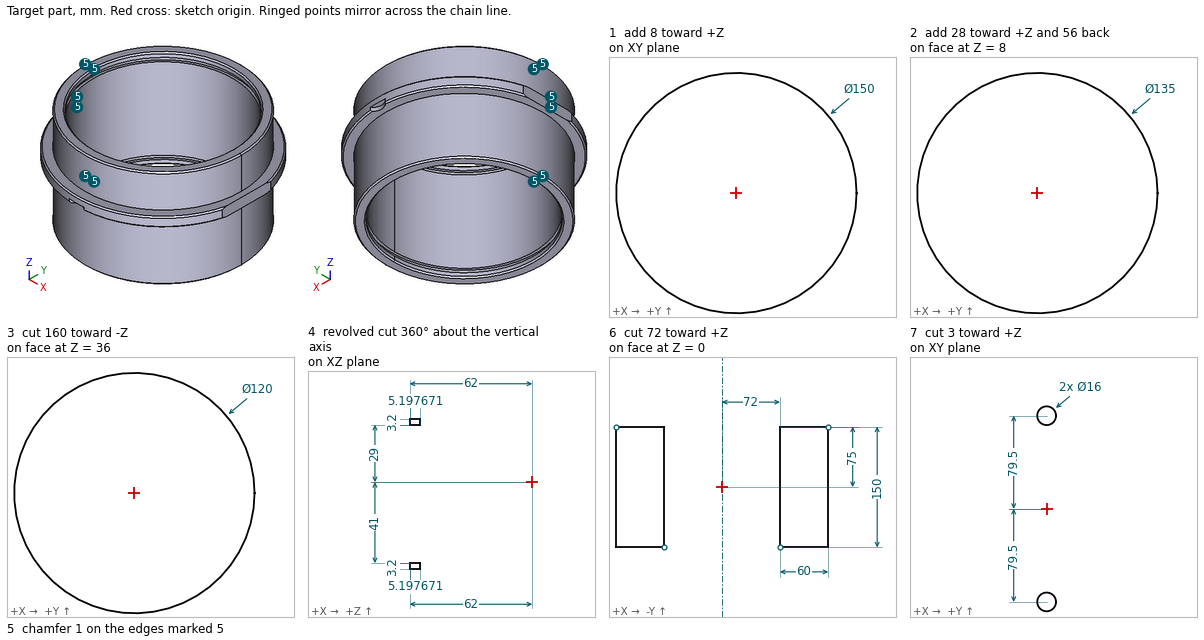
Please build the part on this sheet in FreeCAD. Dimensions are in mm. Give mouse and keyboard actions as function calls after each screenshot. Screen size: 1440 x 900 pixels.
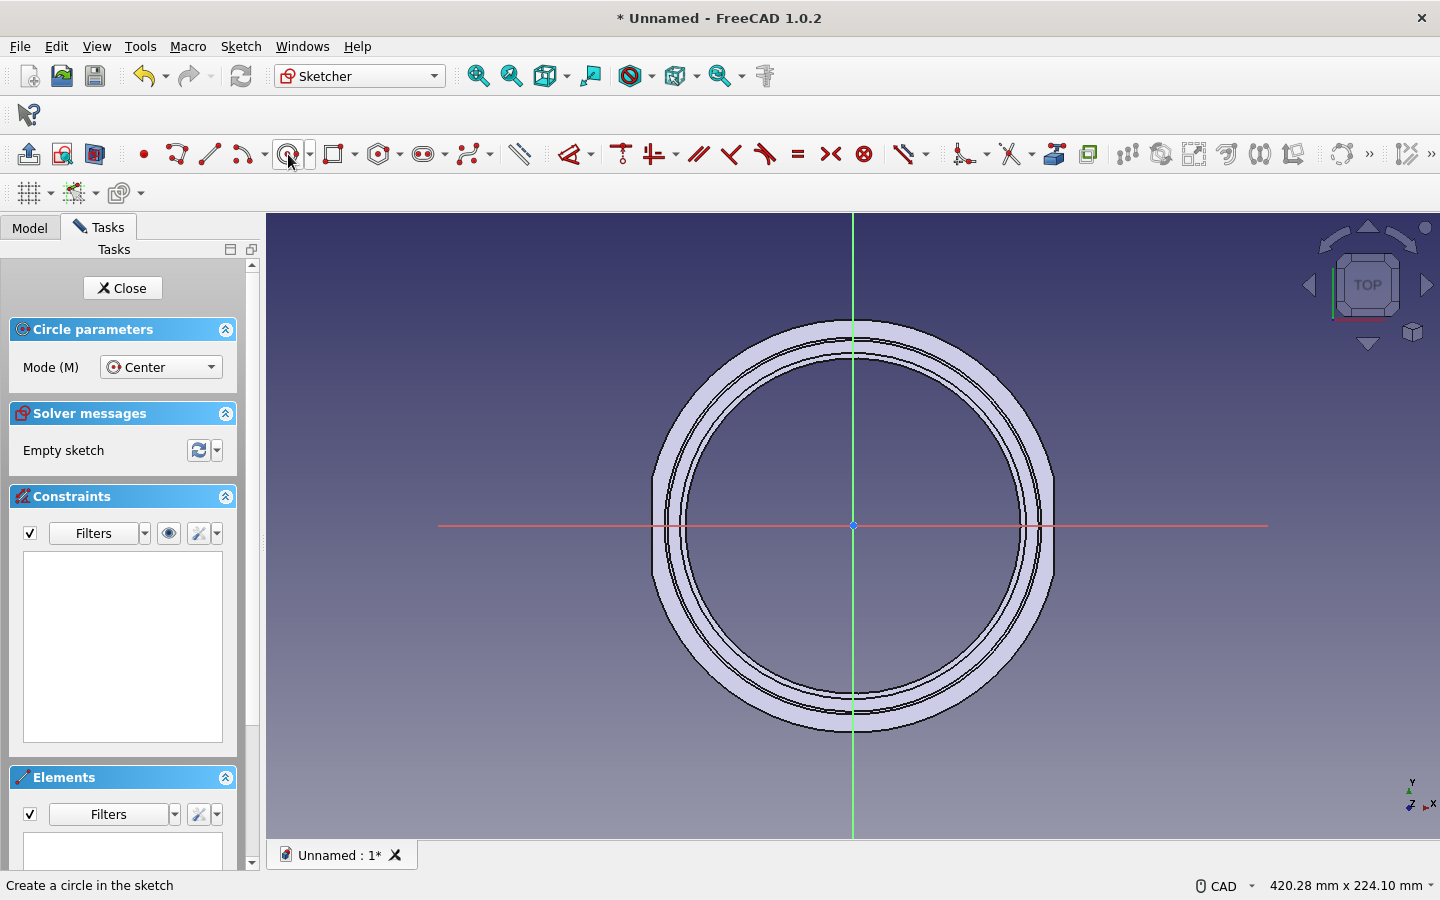
click(853, 304)
click(869, 288)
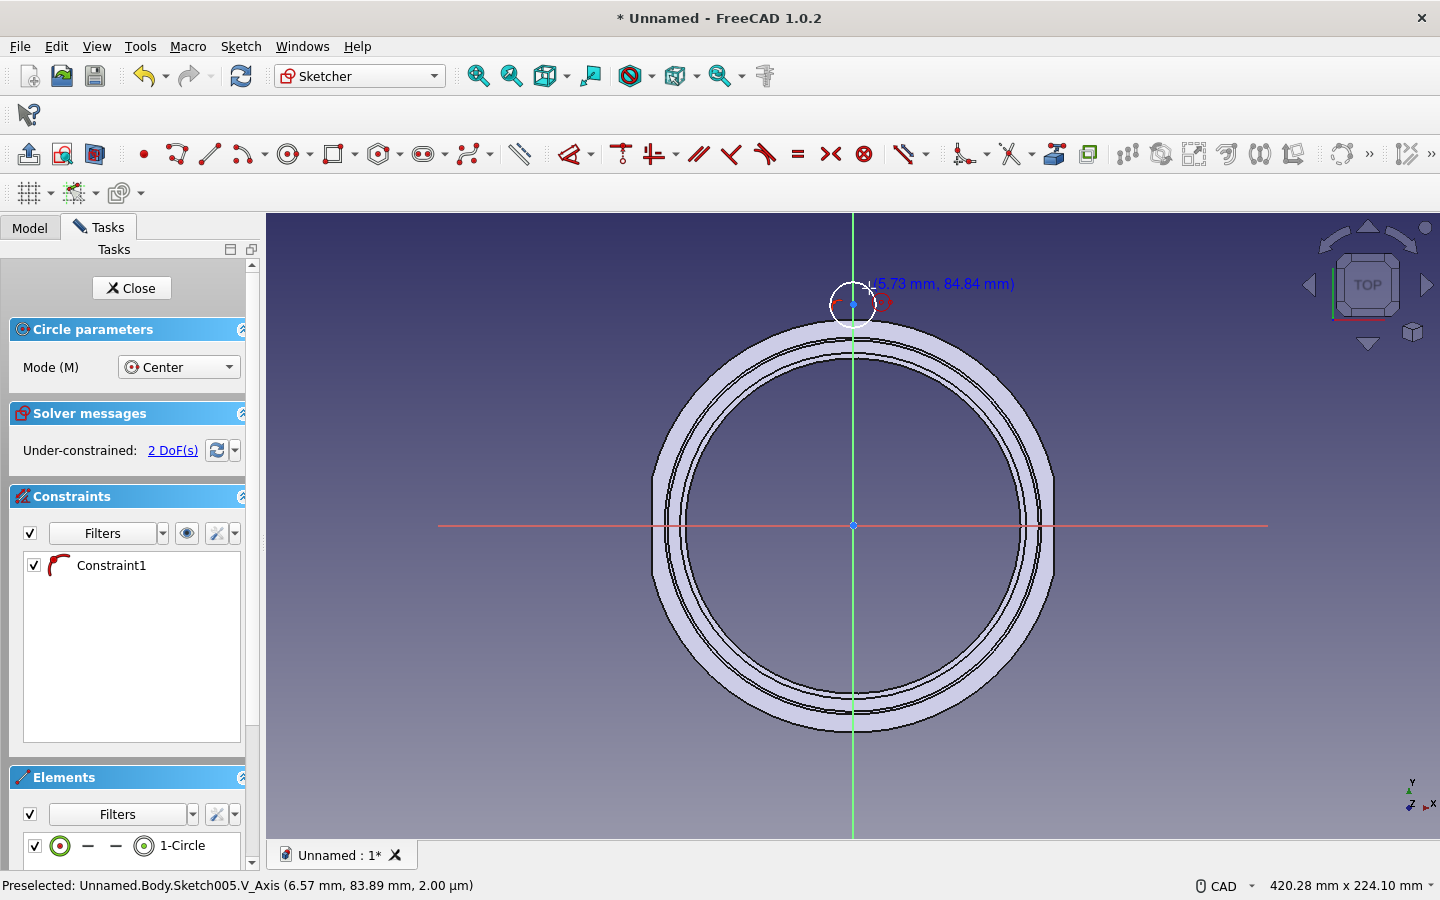
click(853, 748)
click(869, 732)
key(Escape)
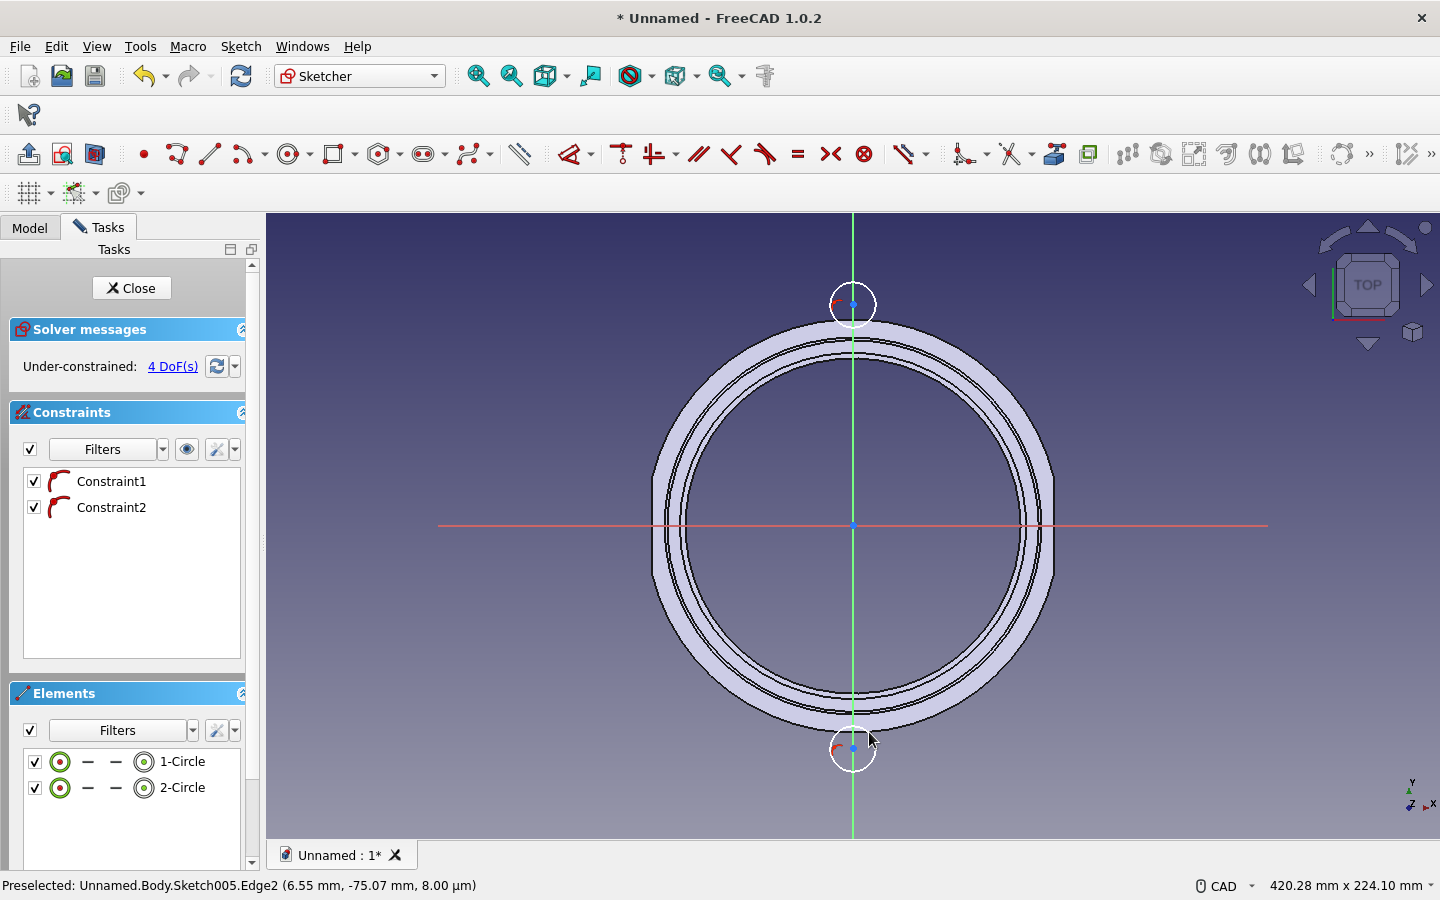
click(869, 289)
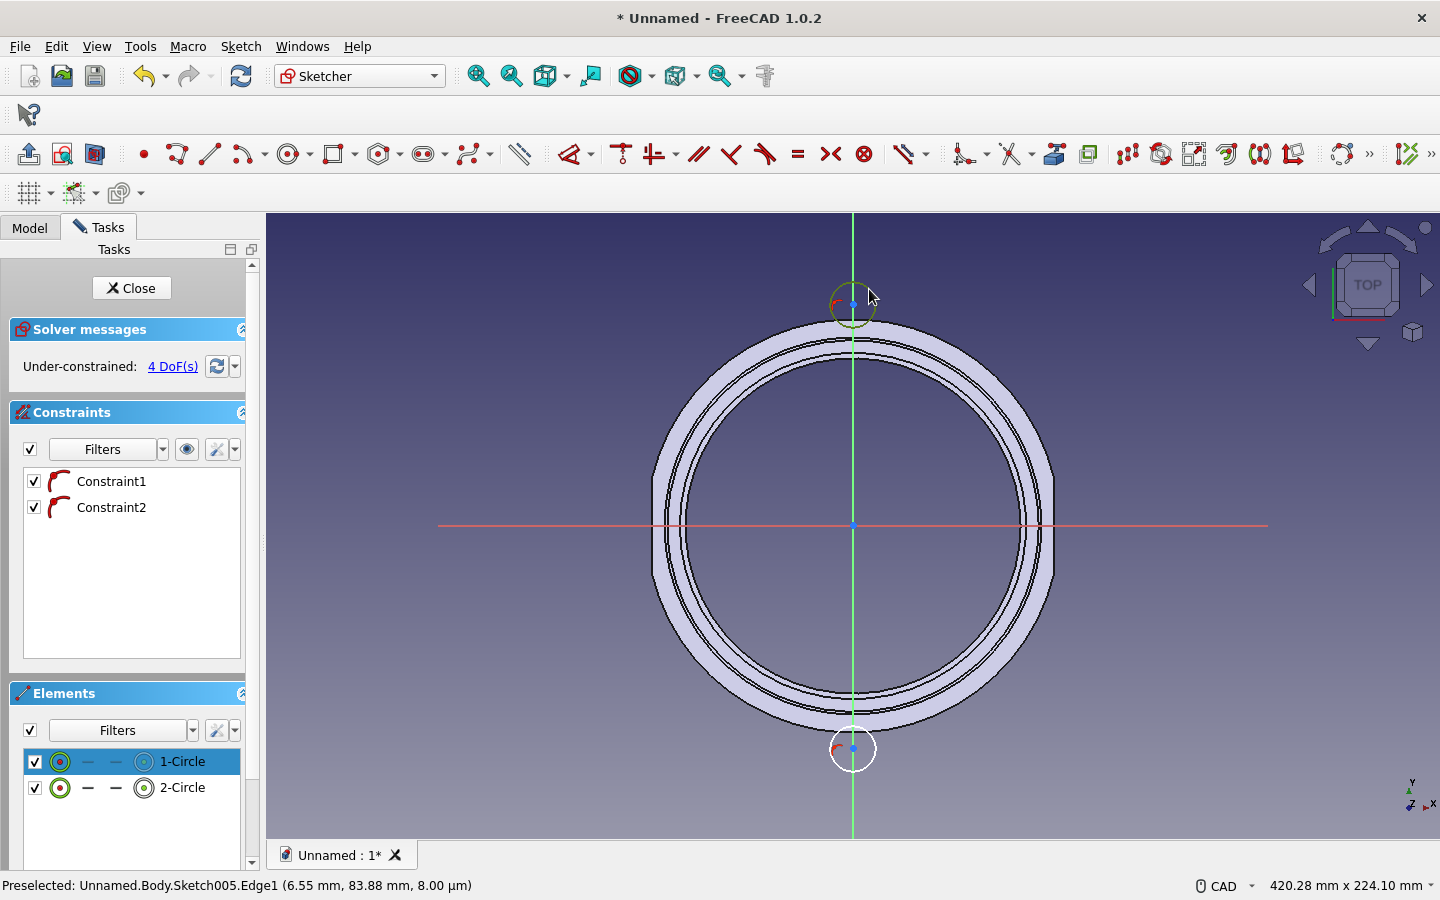
click(869, 733)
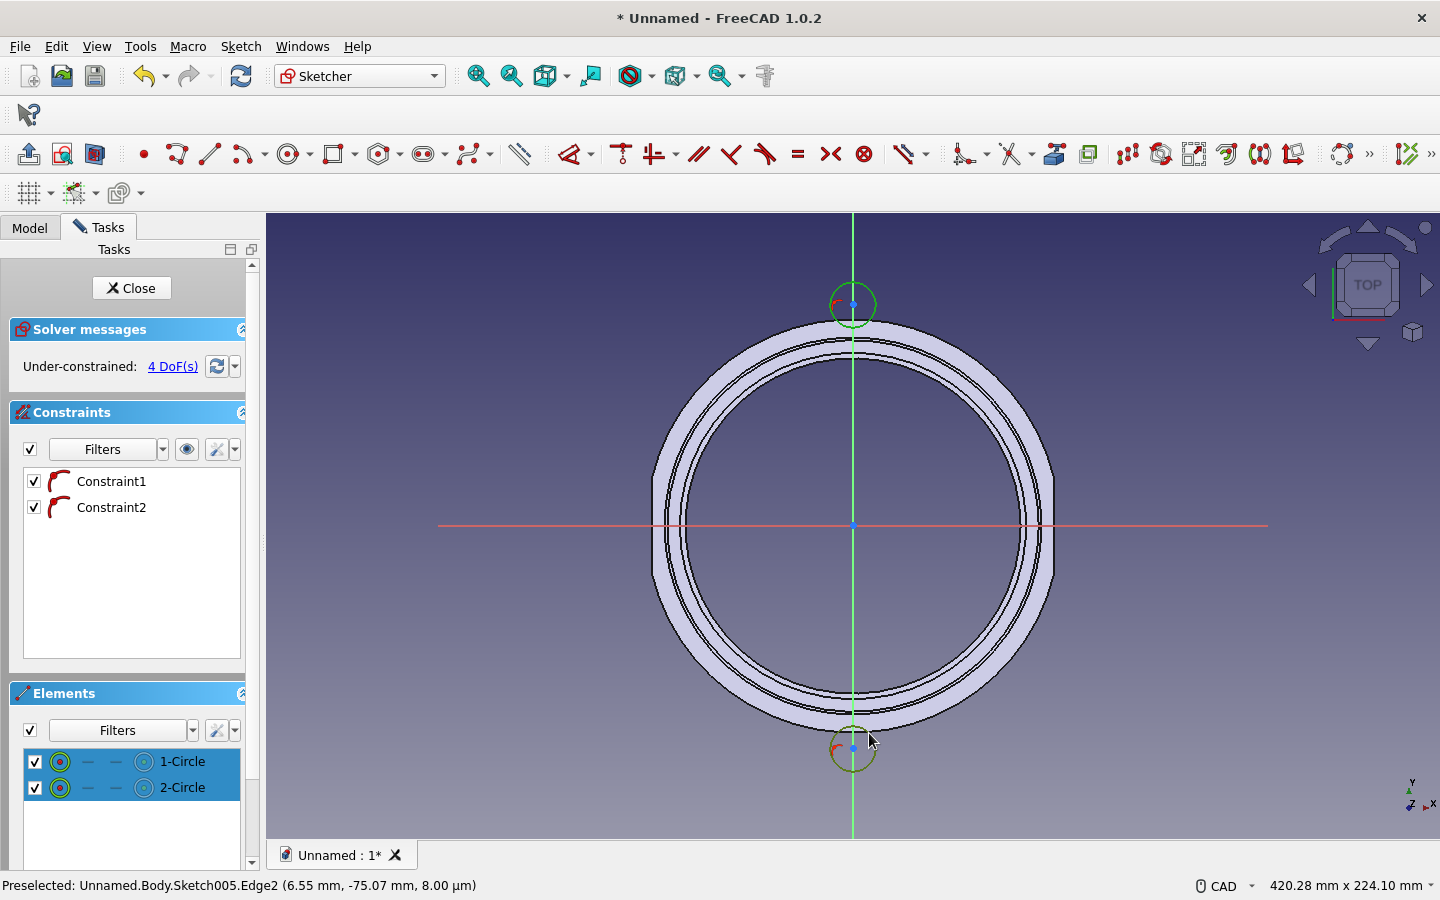
key(e)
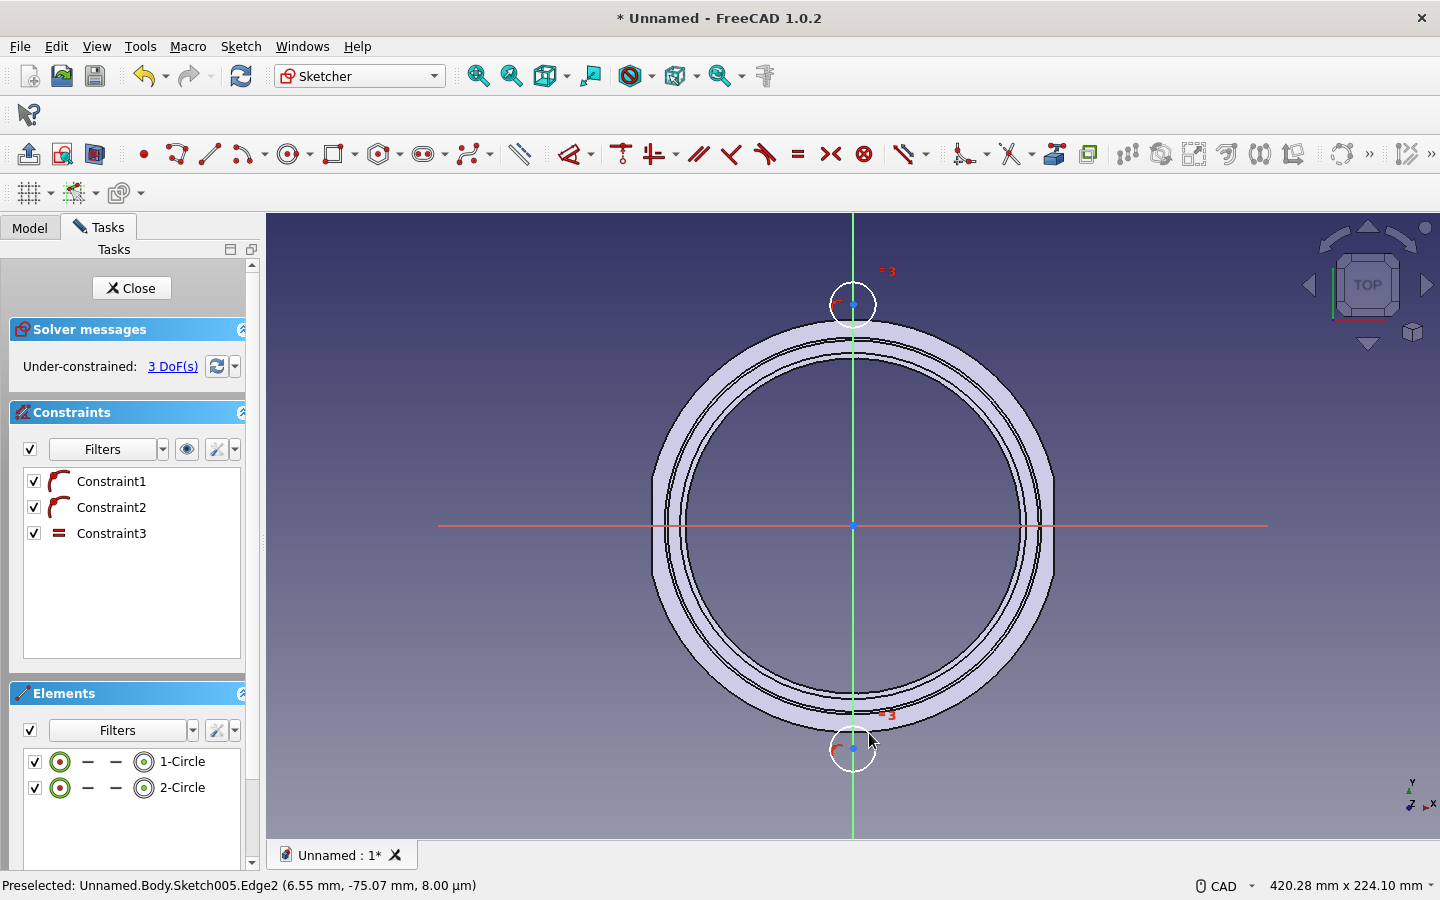
click(568, 154)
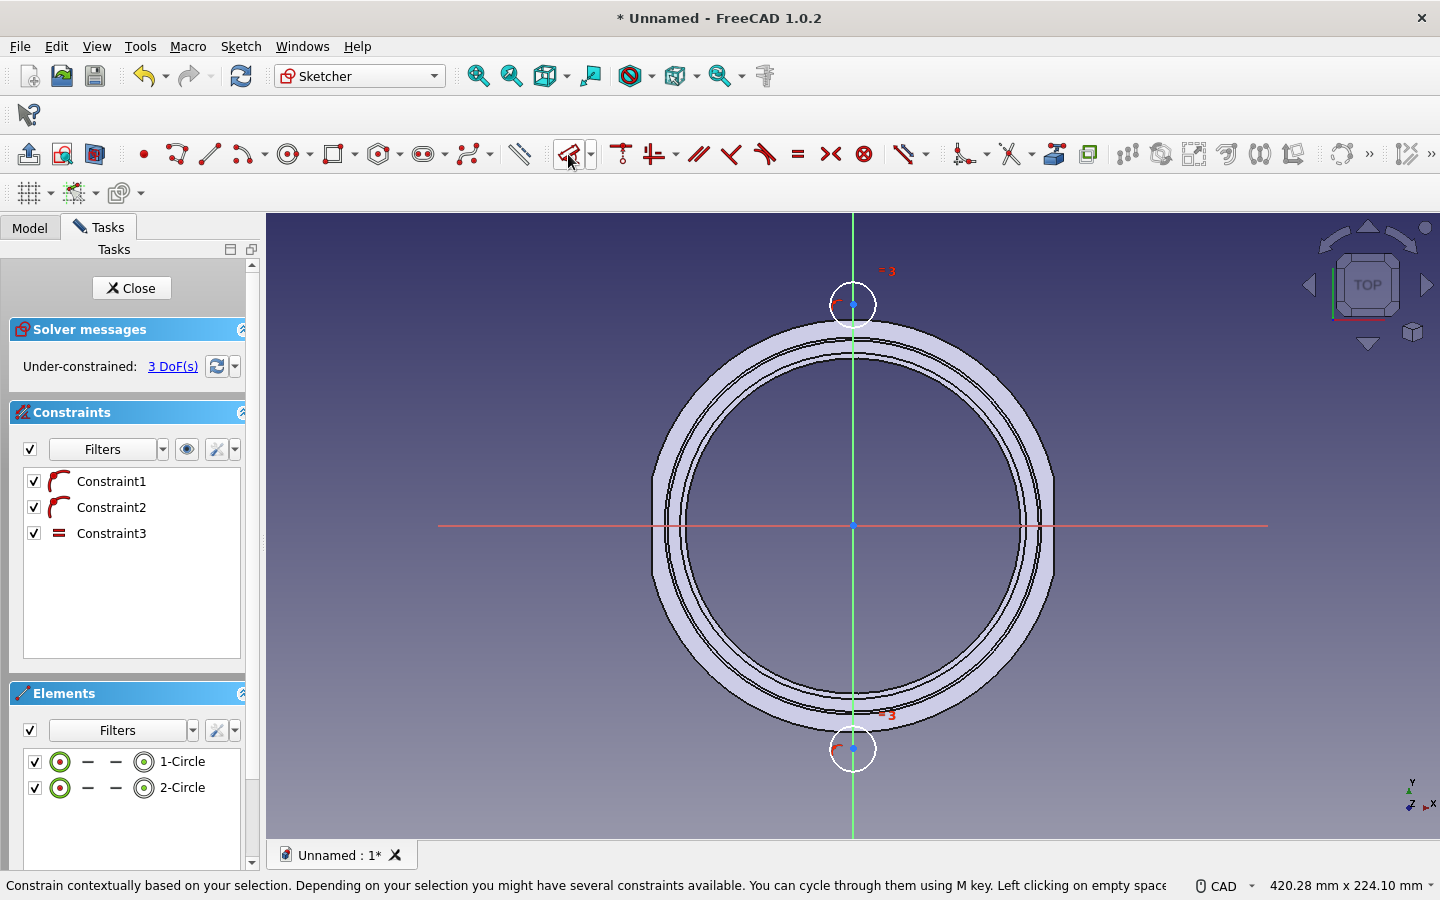
click(869, 289)
click(892, 266)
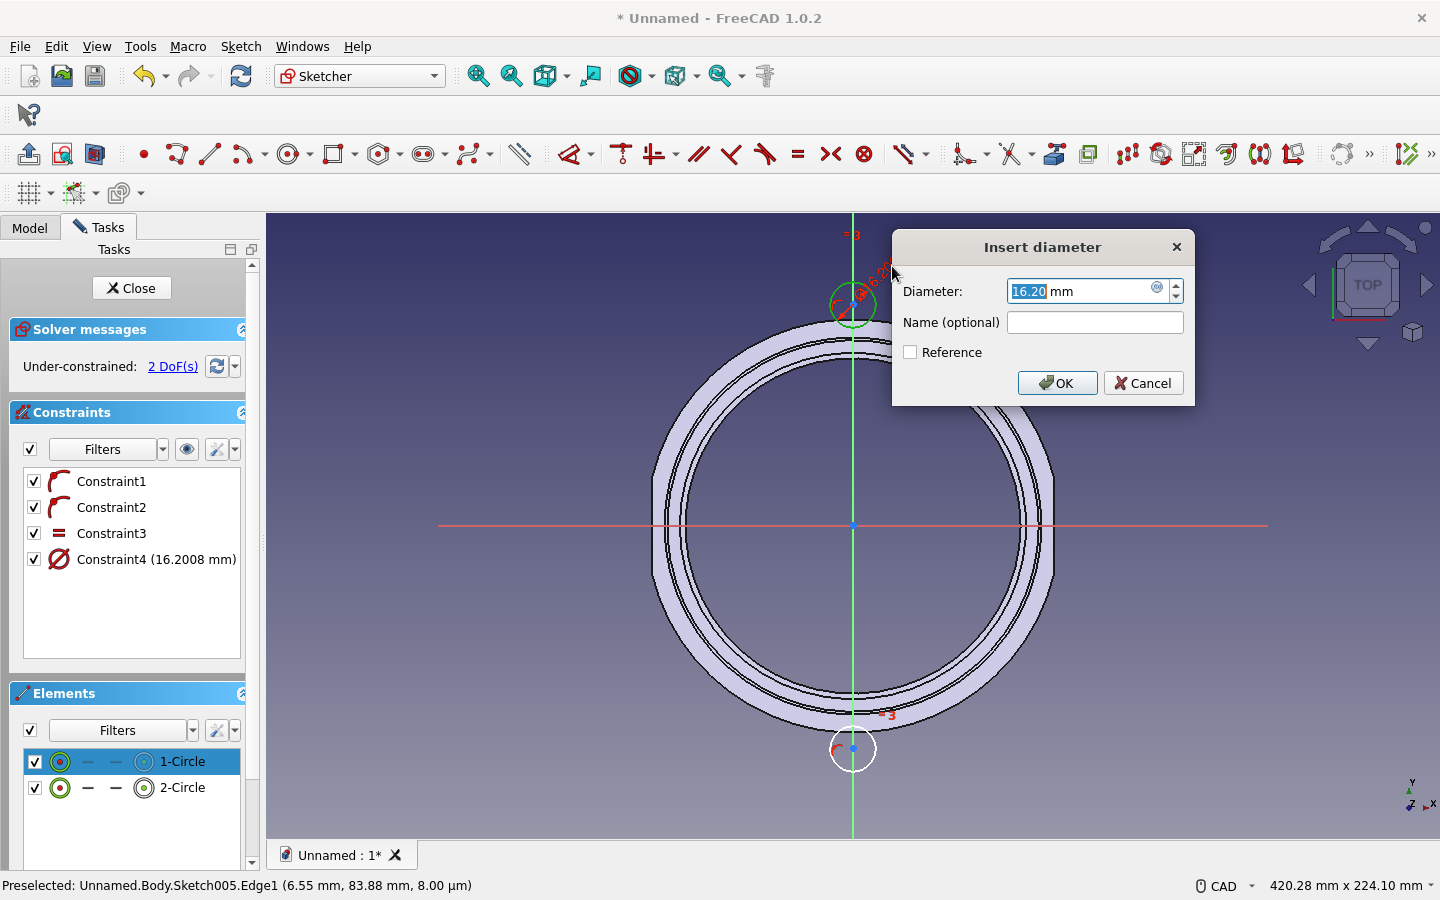
text(16)
key(Return)